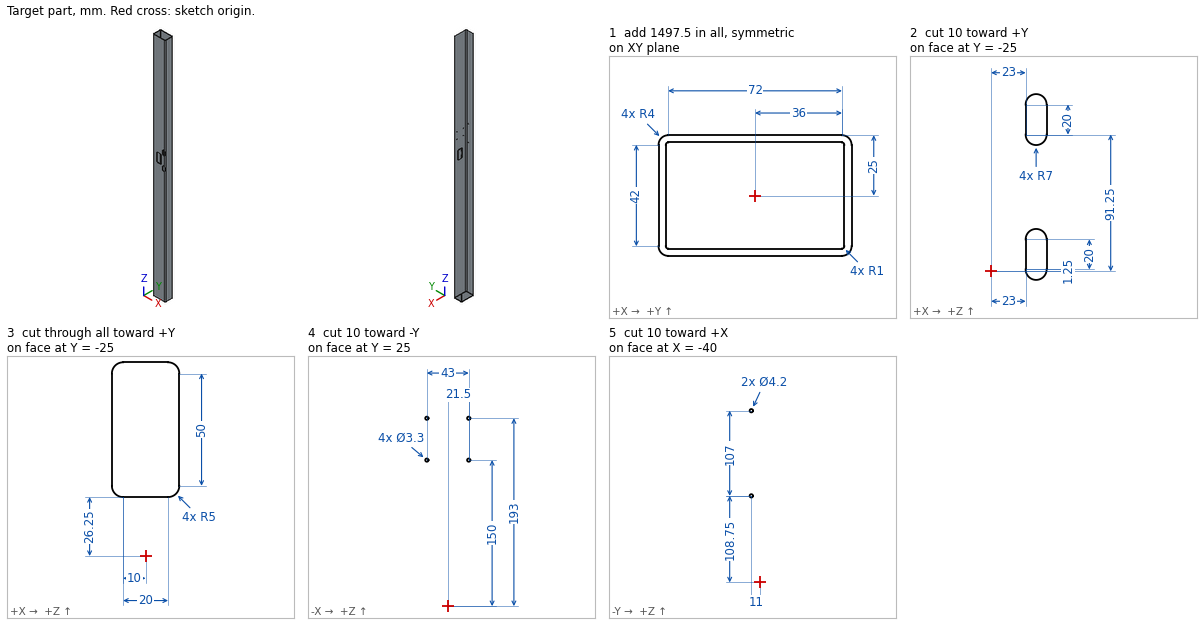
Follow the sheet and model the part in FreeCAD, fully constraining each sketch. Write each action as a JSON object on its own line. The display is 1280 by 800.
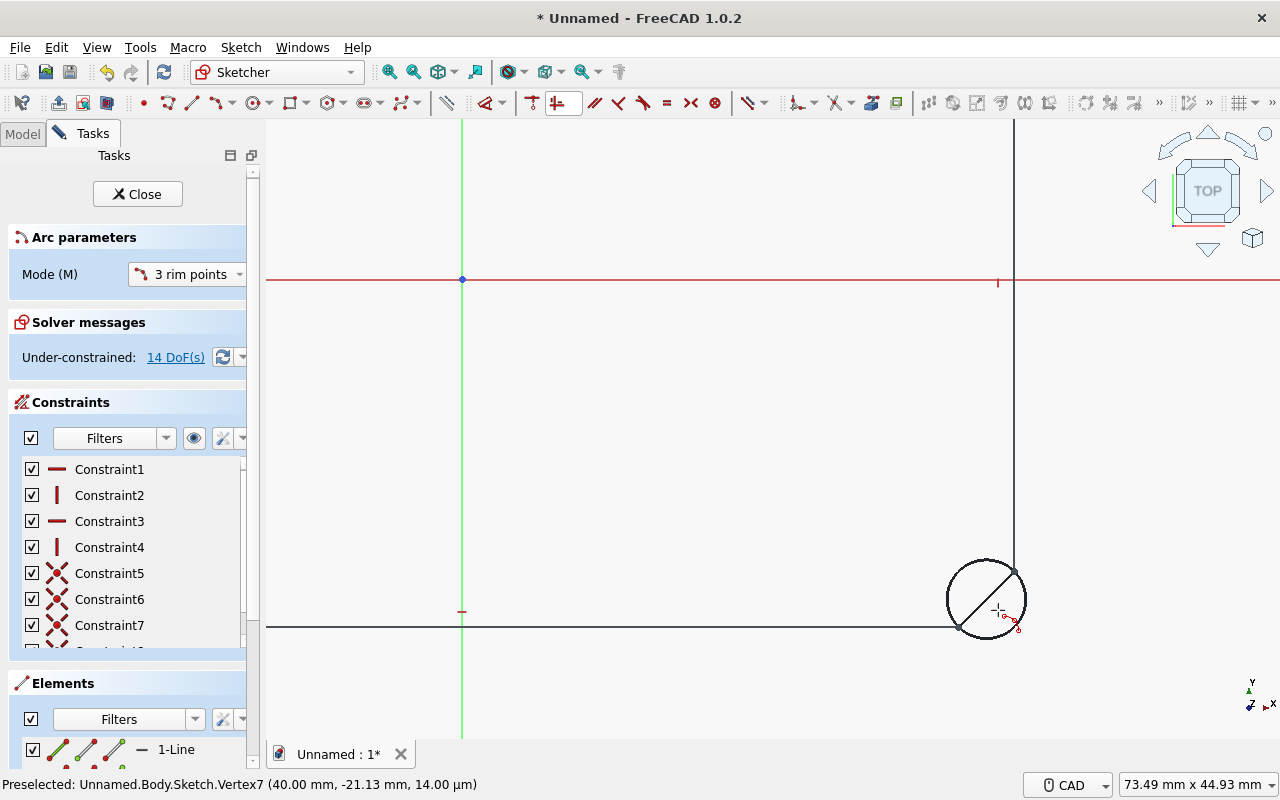
{"action": "left_click", "coordinate": [998, 609]}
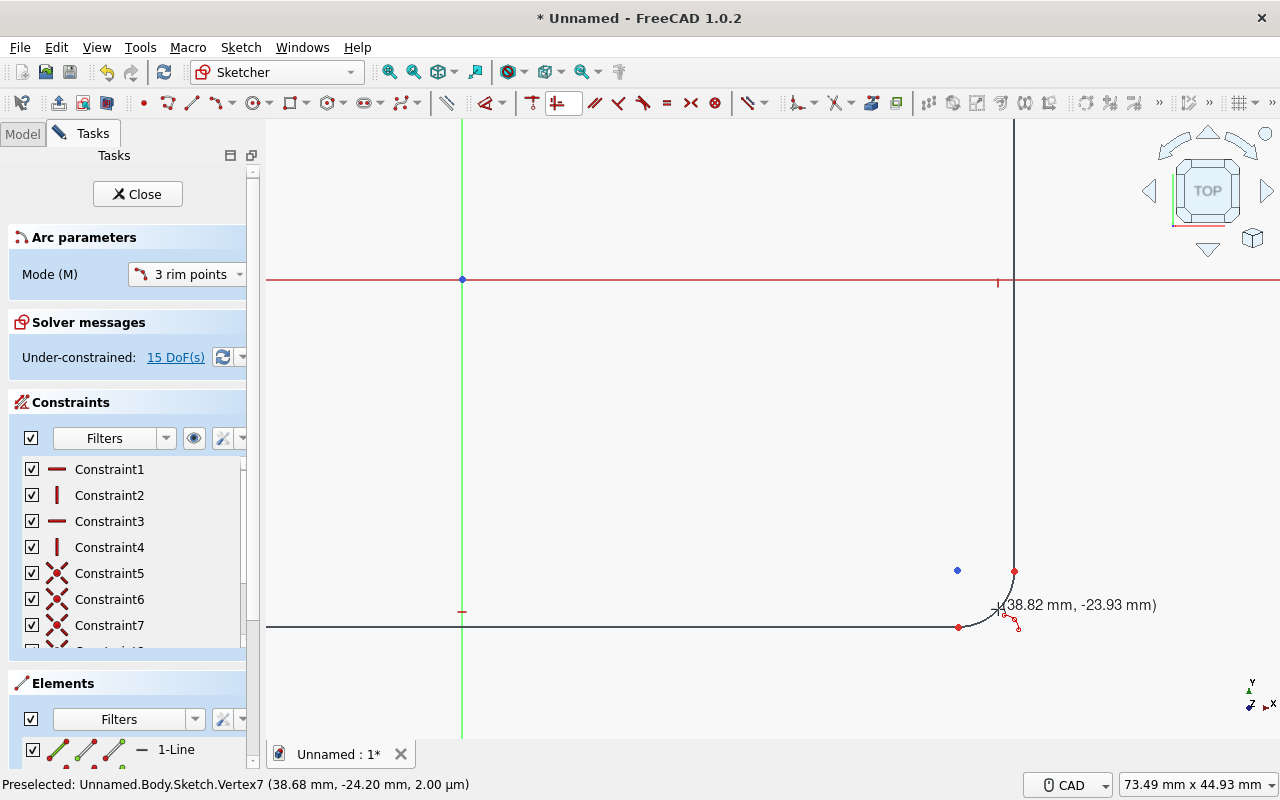
{"action": "scroll", "coordinate": [999, 610], "scroll_direction": "down", "scroll_amount": 3}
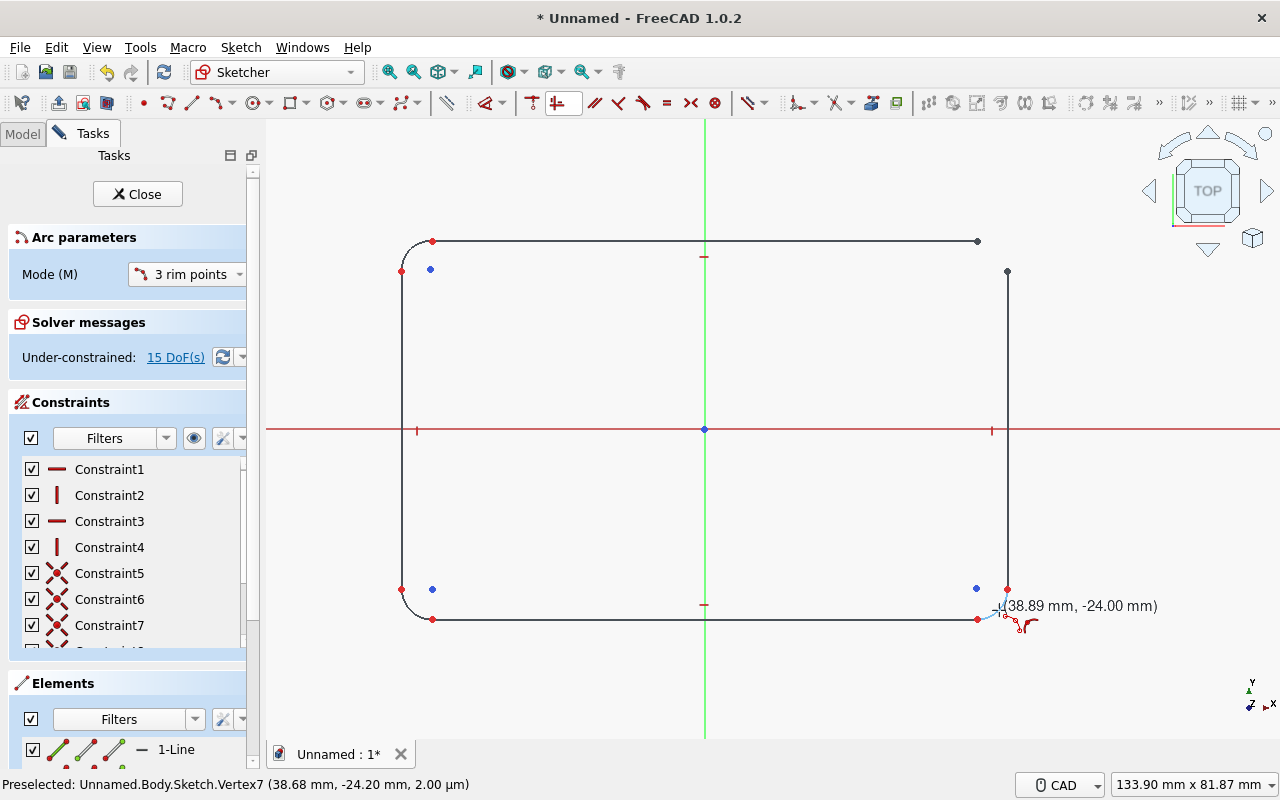
{"action": "left_click", "coordinate": [1008, 272]}
{"action": "left_click", "coordinate": [977, 241]}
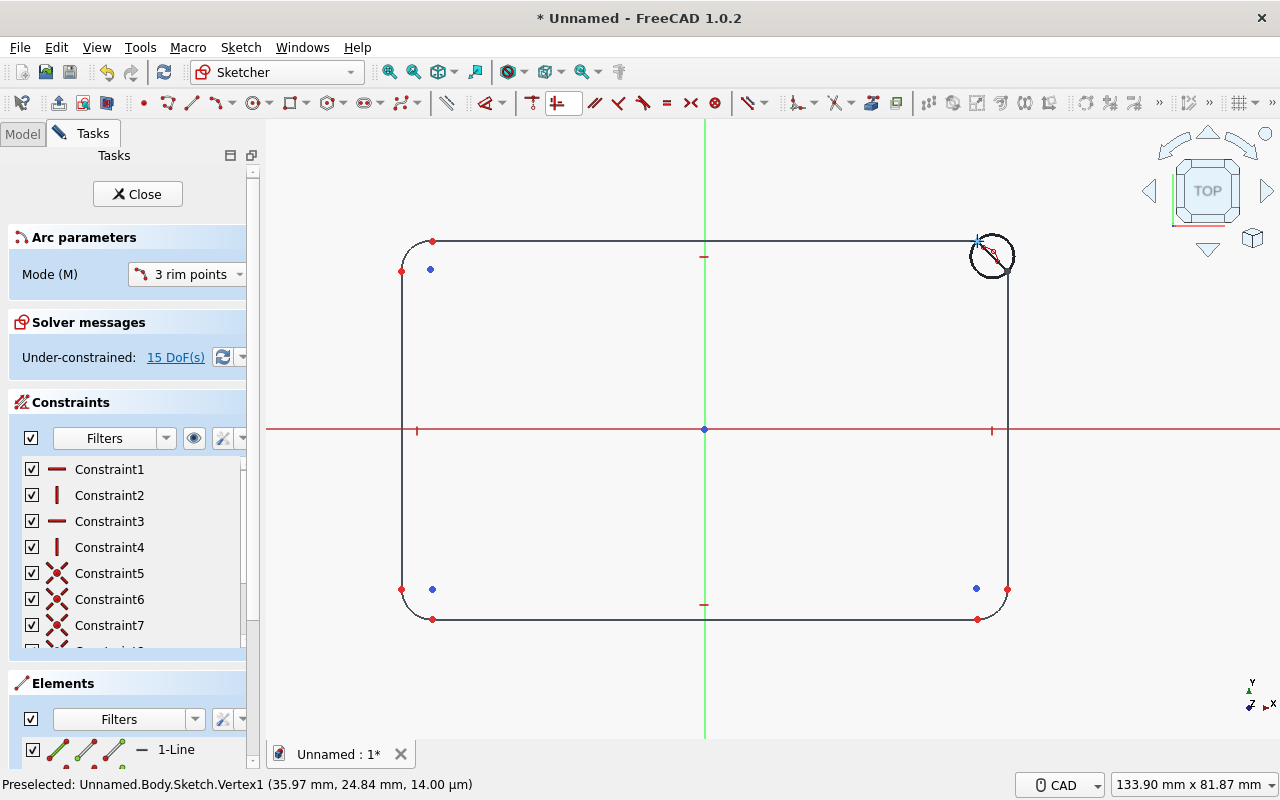
{"action": "scroll", "coordinate": [999, 249], "scroll_direction": "up", "scroll_amount": 3}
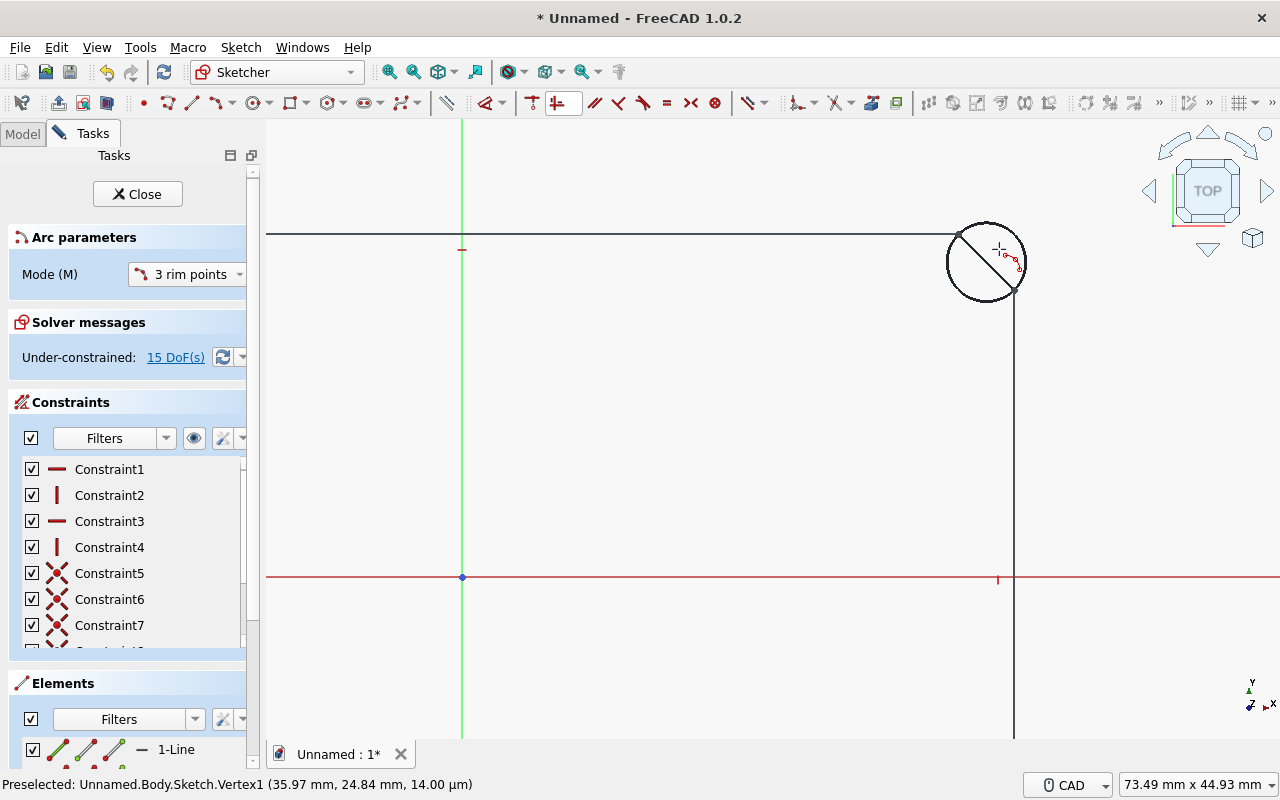
{"action": "left_click", "coordinate": [998, 248]}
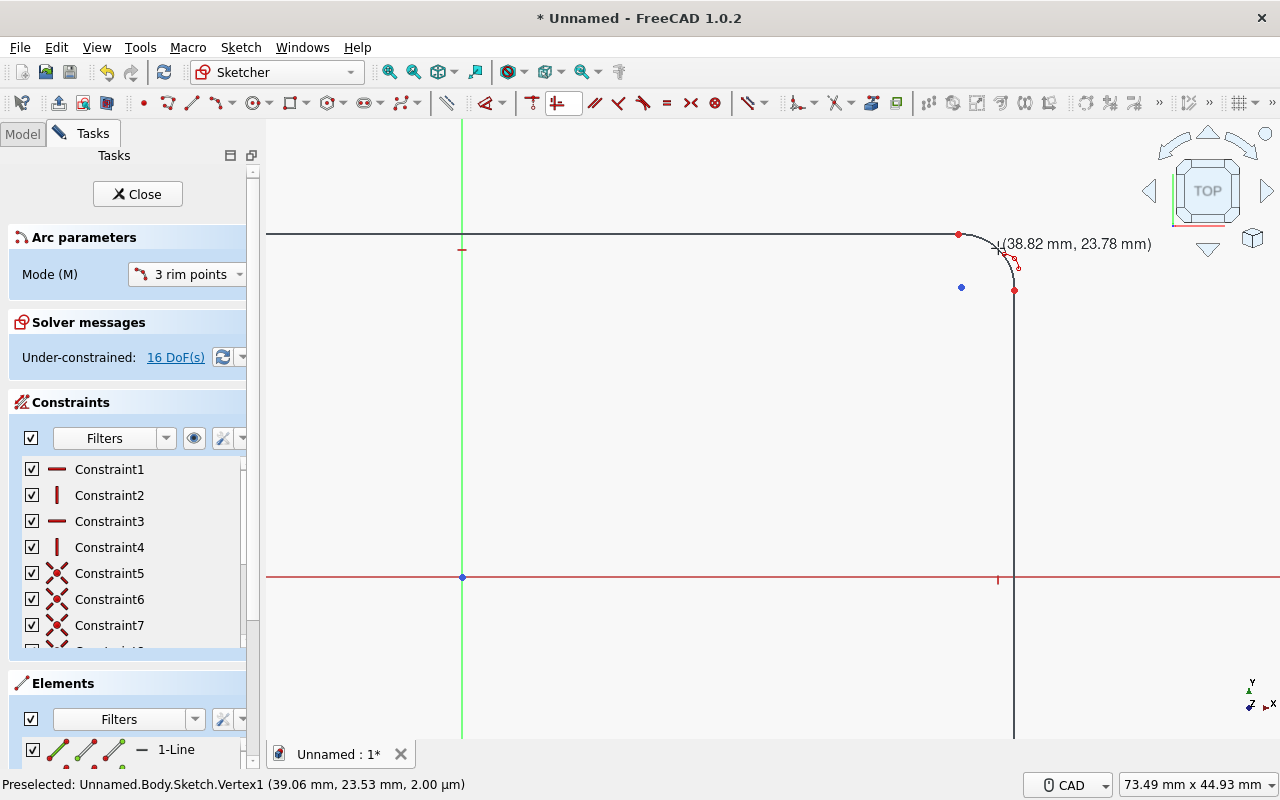
{"action": "left_click", "coordinate": [192, 104]}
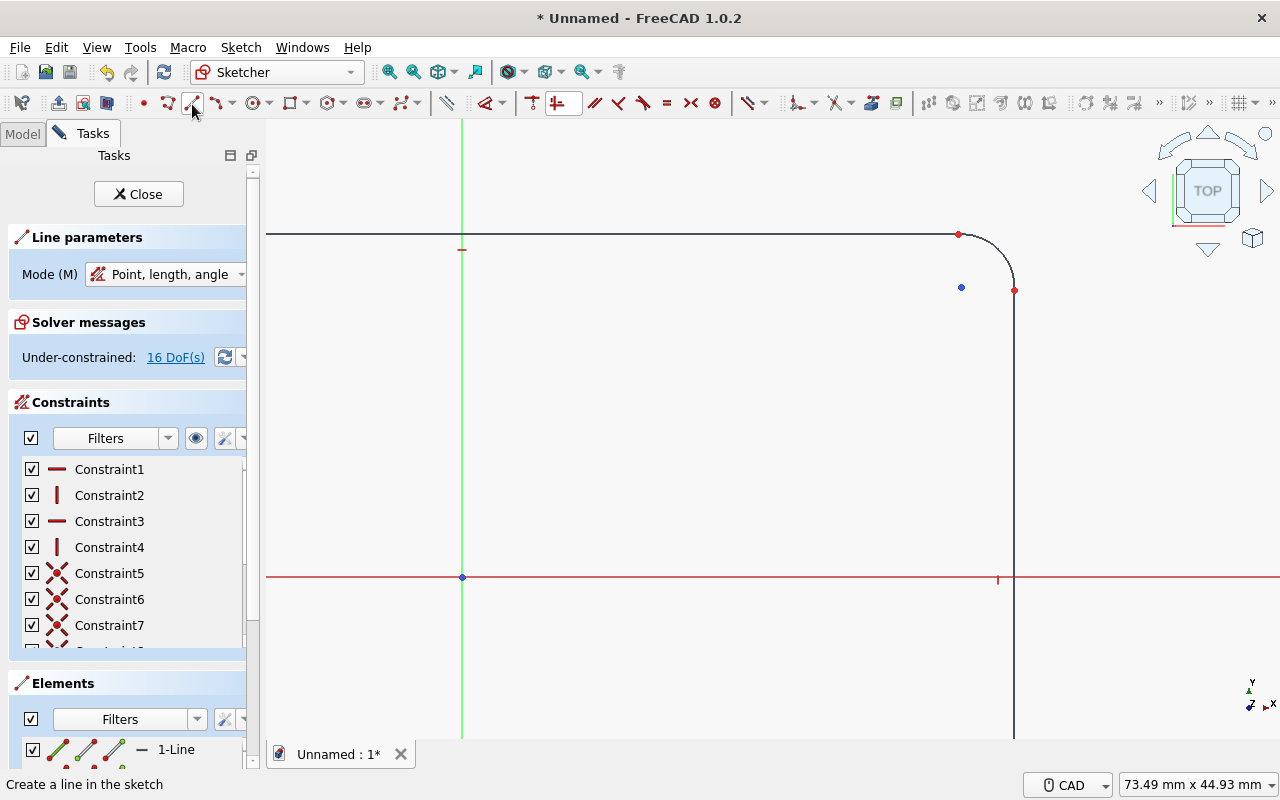
{"action": "scroll", "coordinate": [999, 249], "scroll_direction": "down", "scroll_amount": 3}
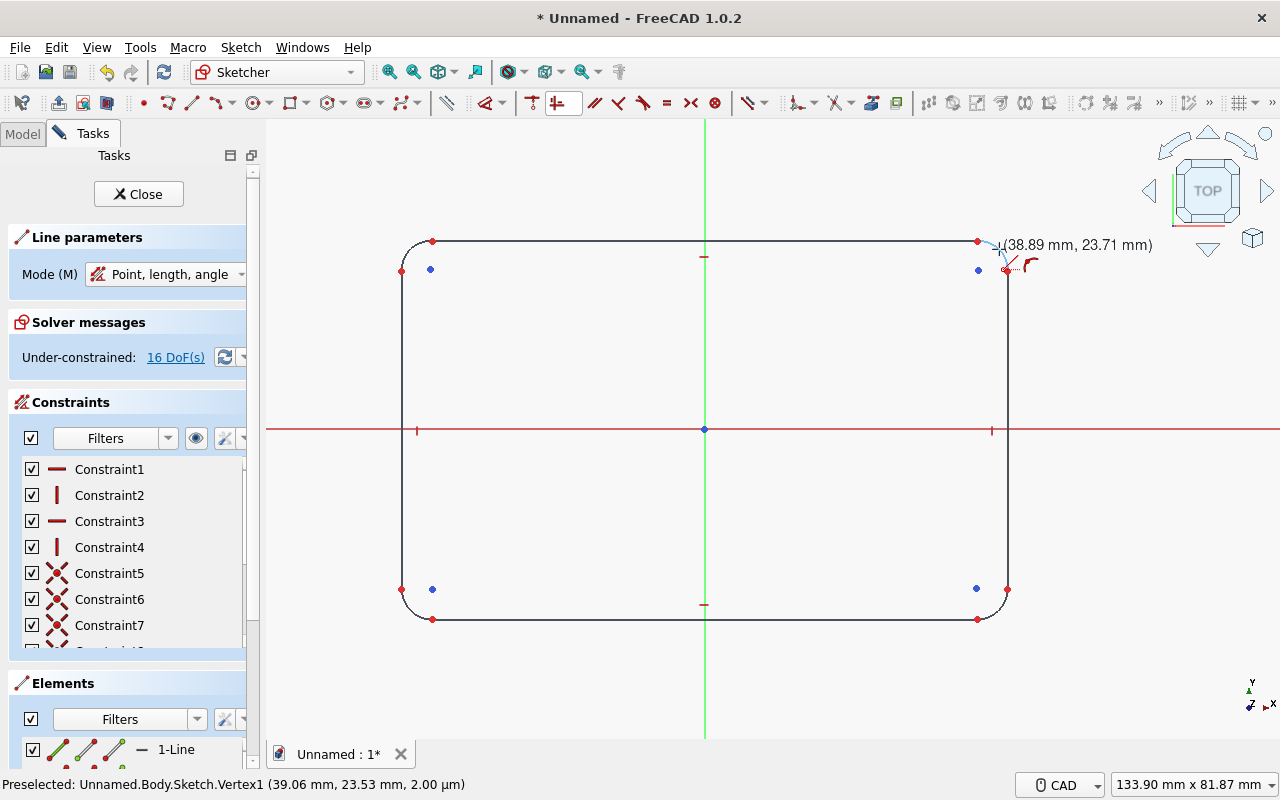
{"action": "scroll", "coordinate": [432, 263], "scroll_direction": "up", "scroll_amount": 4}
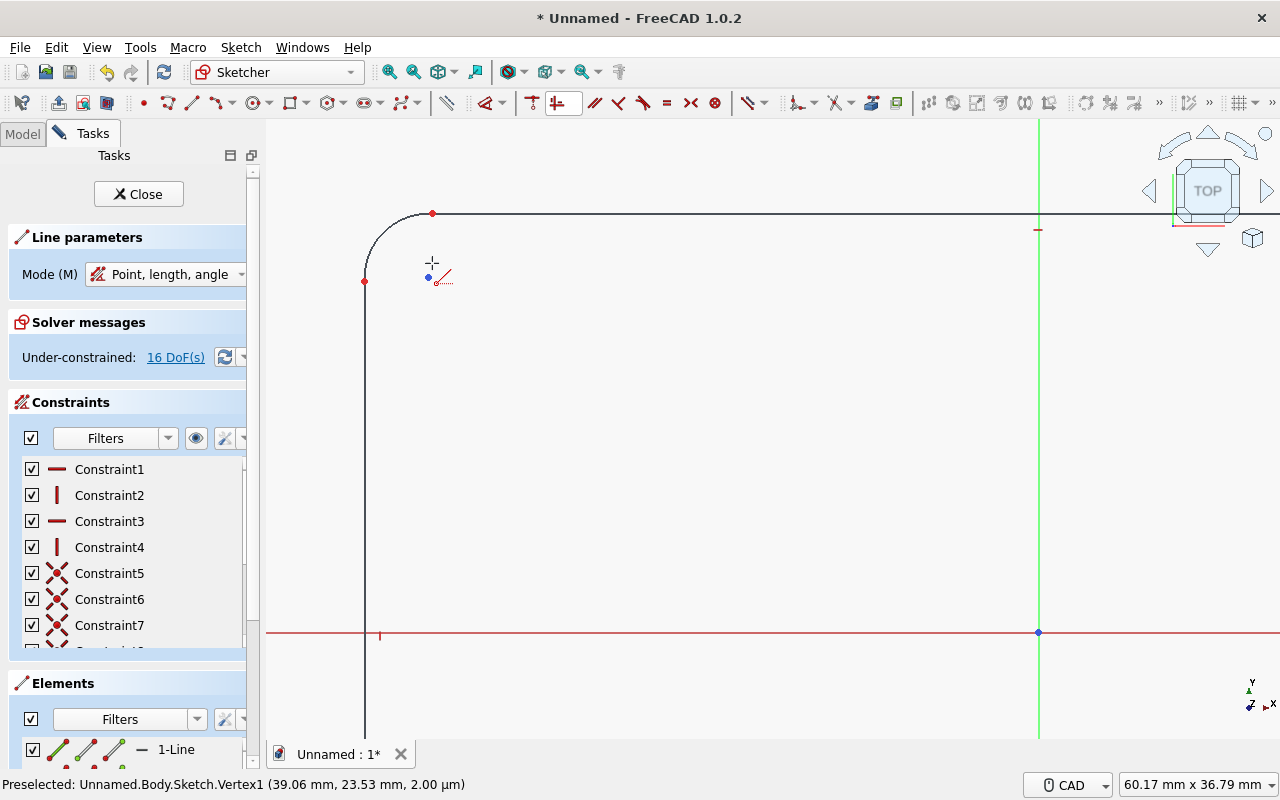
{"action": "left_click", "coordinate": [432, 262]}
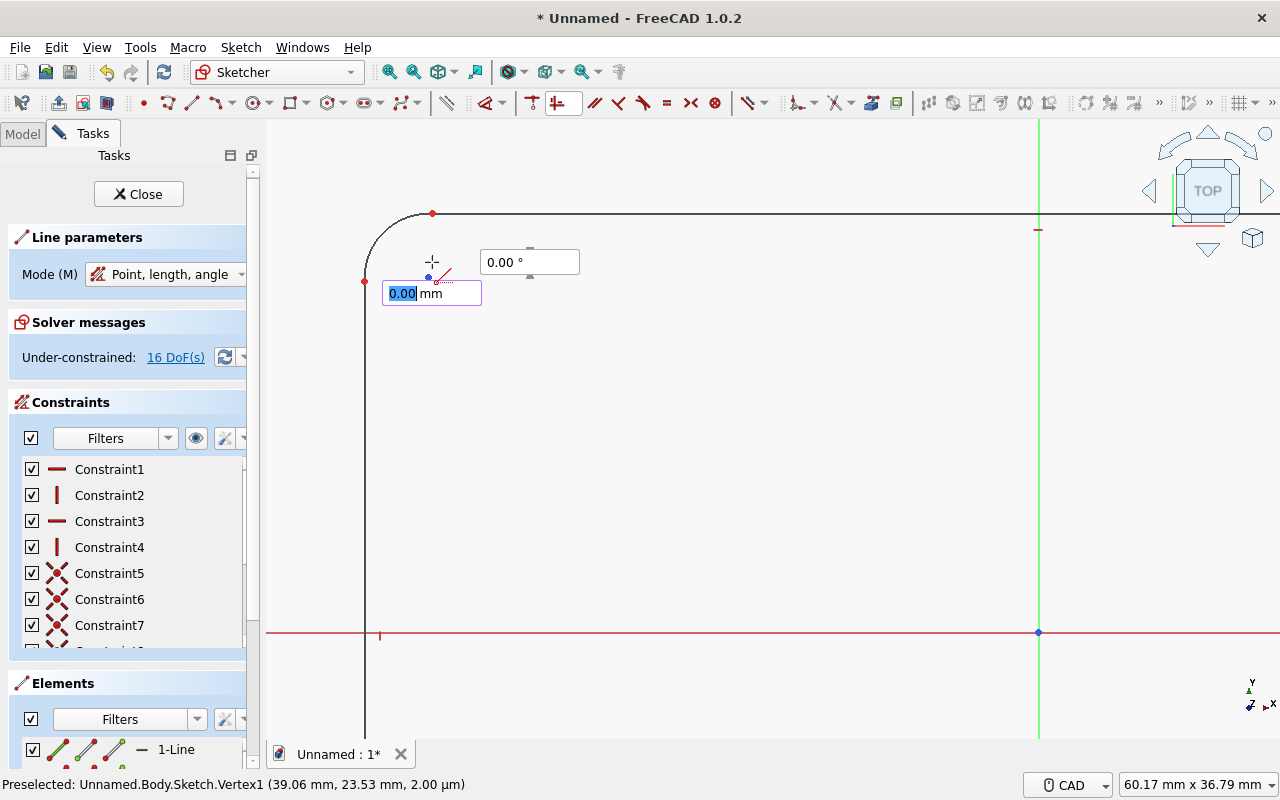
{"action": "scroll", "coordinate": [432, 263], "scroll_direction": "down", "scroll_amount": 4}